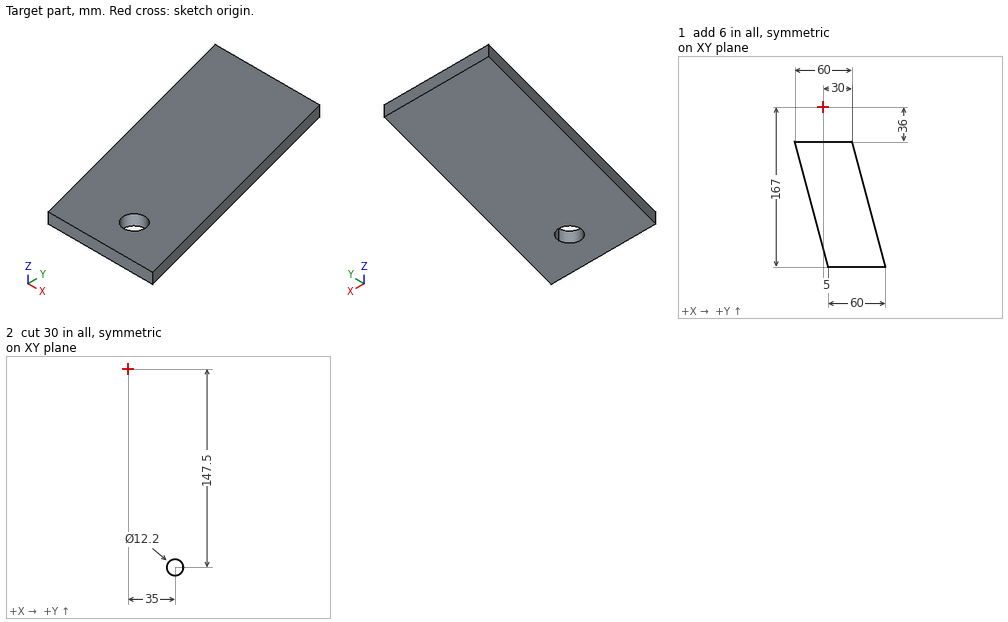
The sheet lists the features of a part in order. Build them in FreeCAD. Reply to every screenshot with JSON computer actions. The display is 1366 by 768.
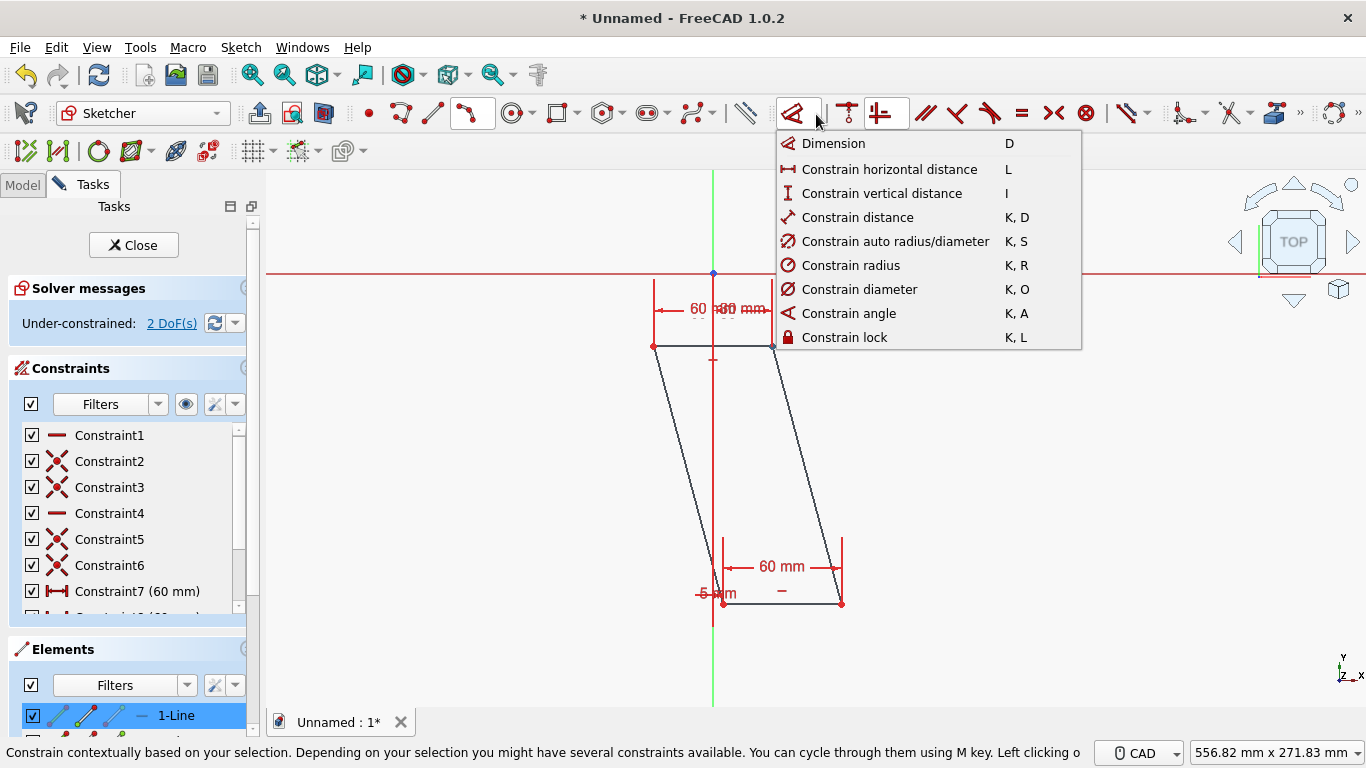
{"action": "left_click", "coordinate": [929, 193]}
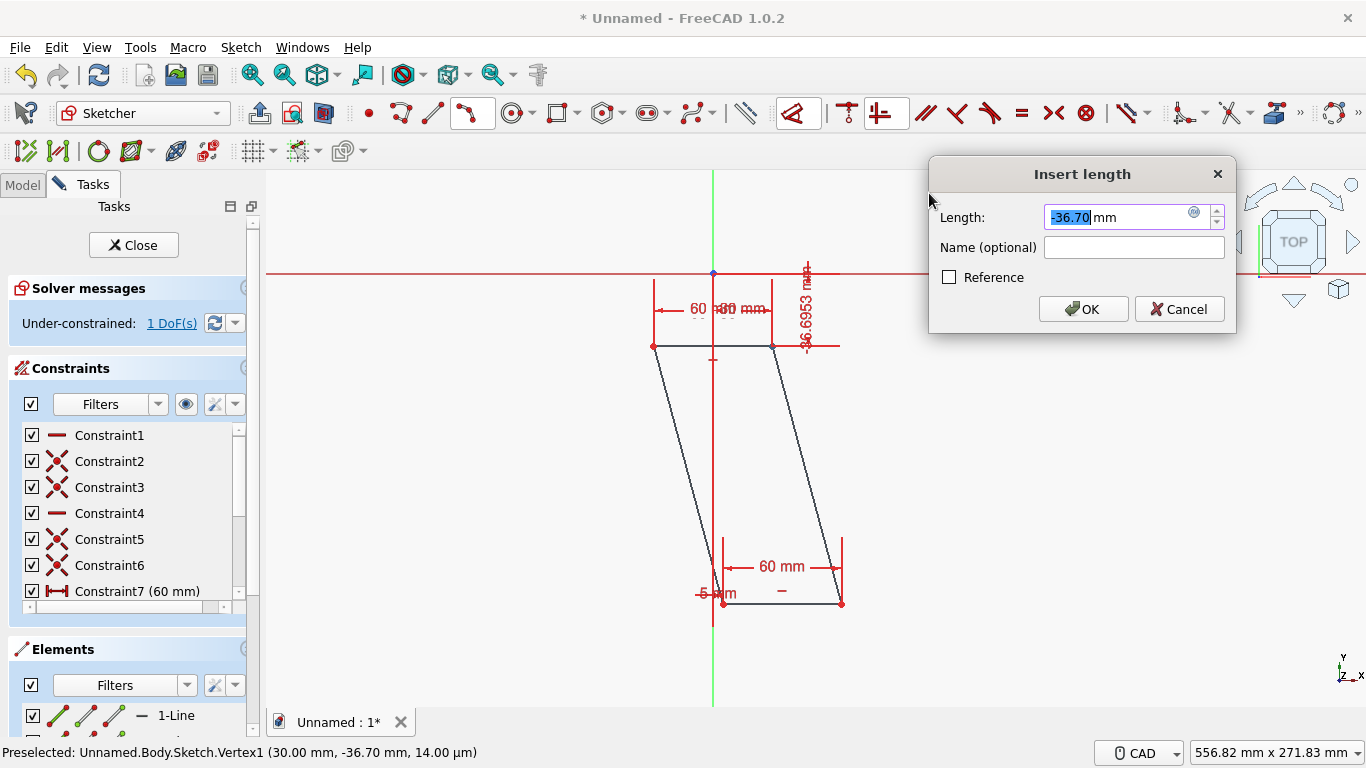
{"action": "type", "text": "-36"}
{"action": "key", "text": "Return"}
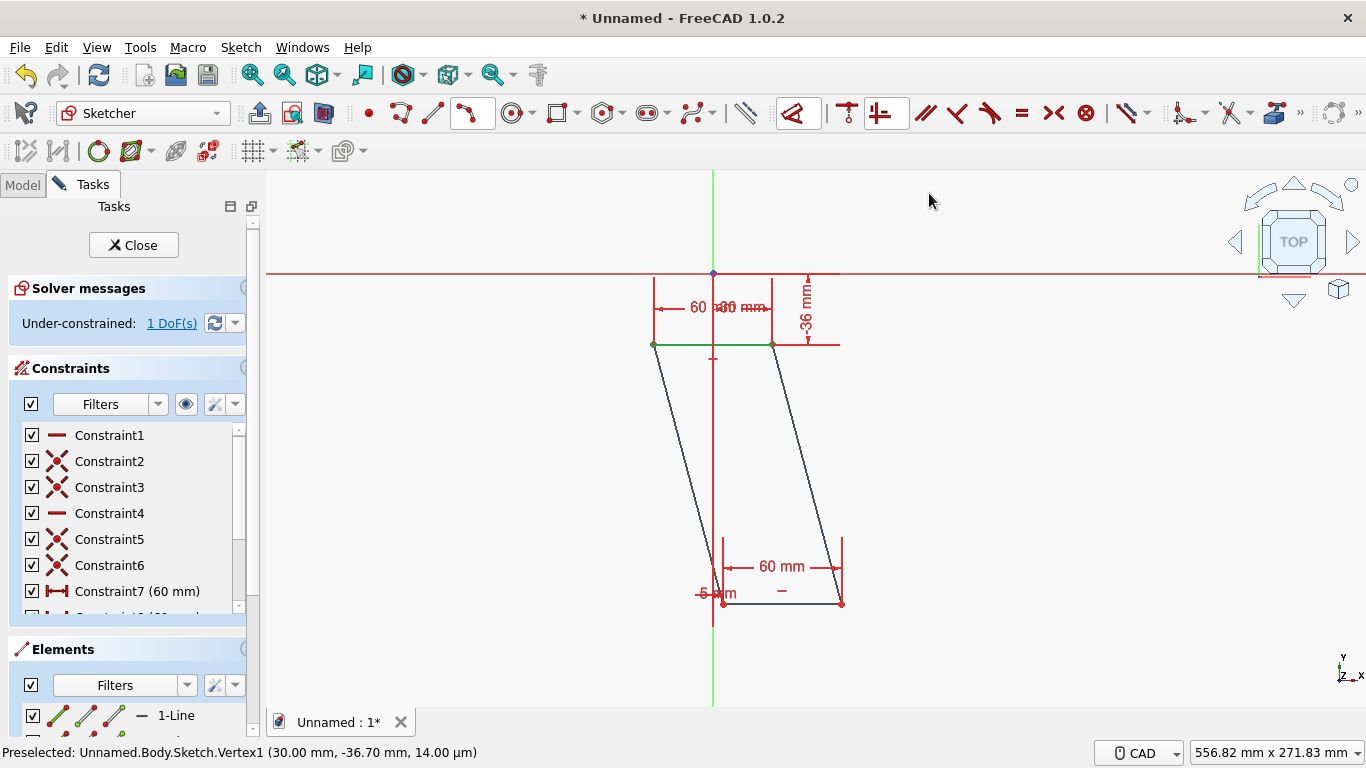
{"action": "left_click", "coordinate": [723, 604]}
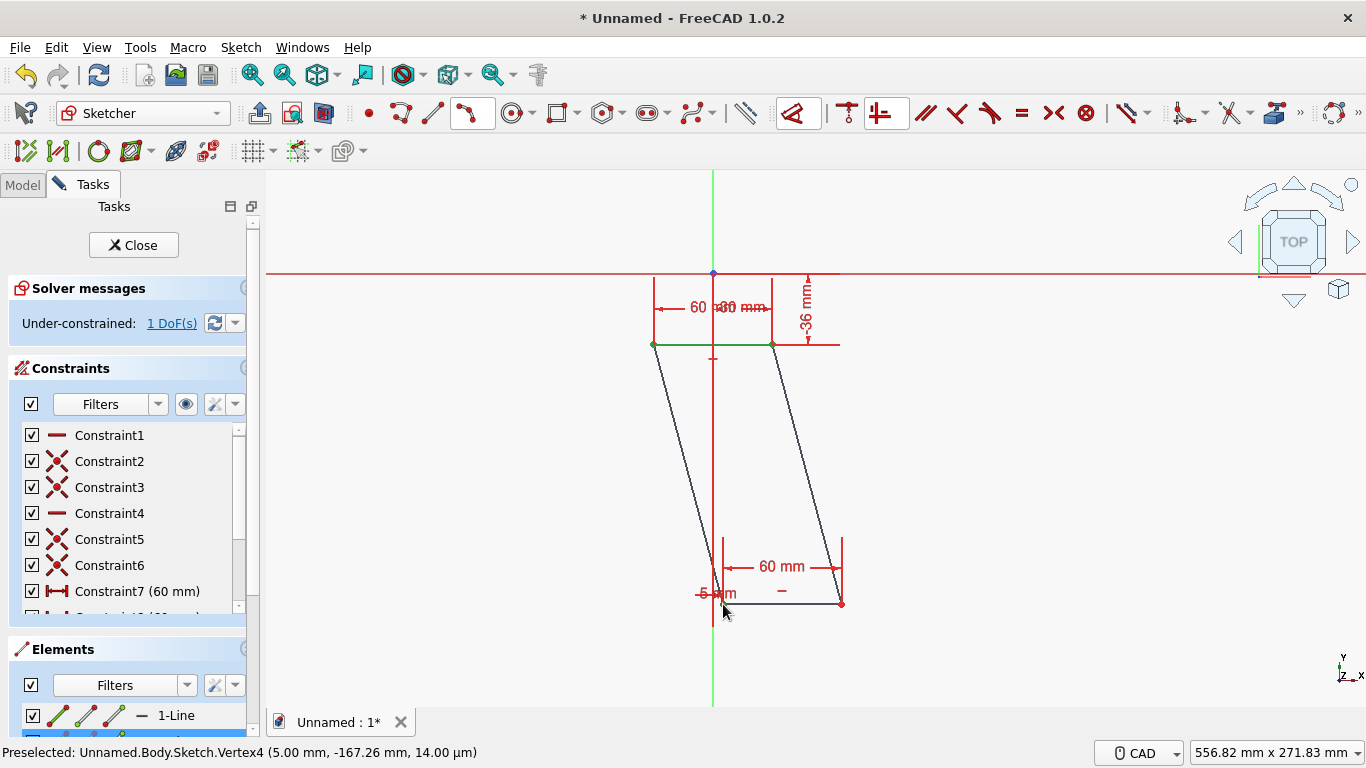
{"action": "key", "text": "i"}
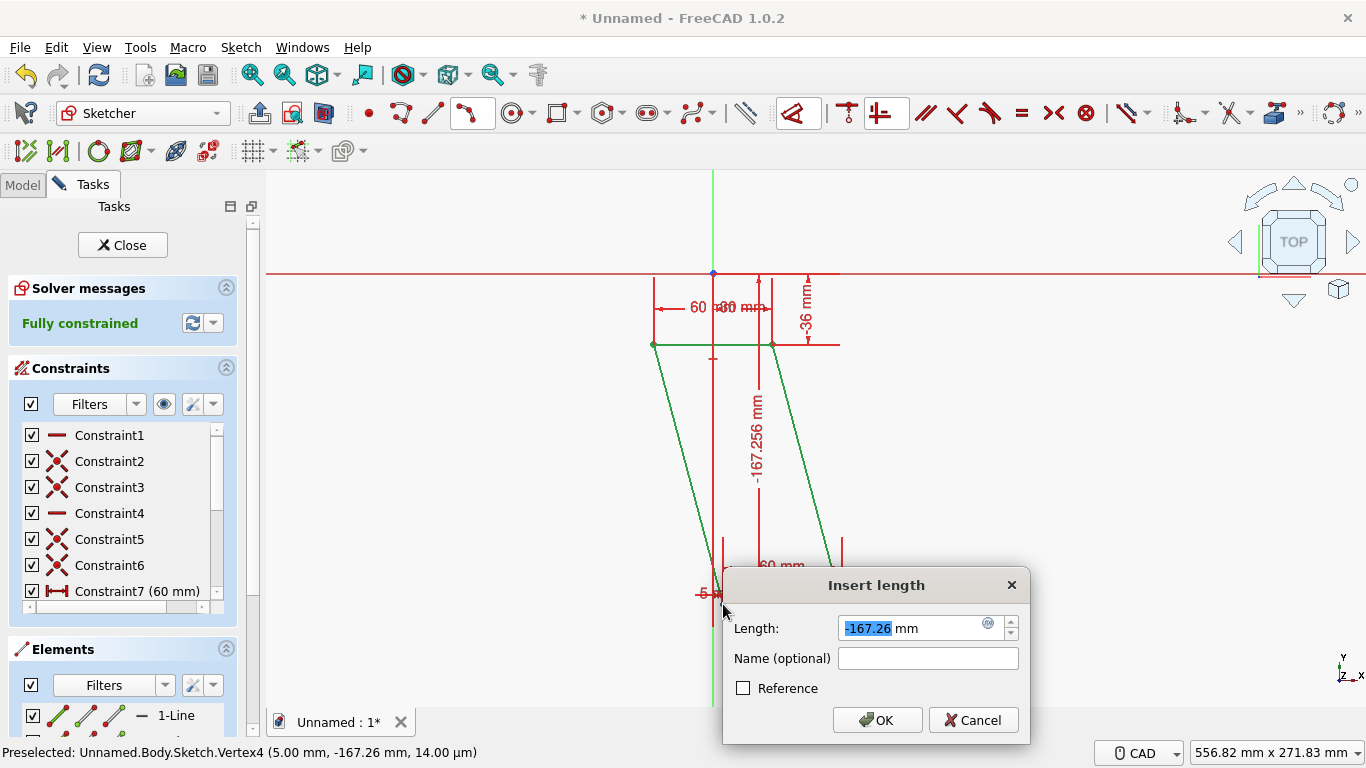
{"action": "type", "text": "-167"}
{"action": "key", "text": "Return"}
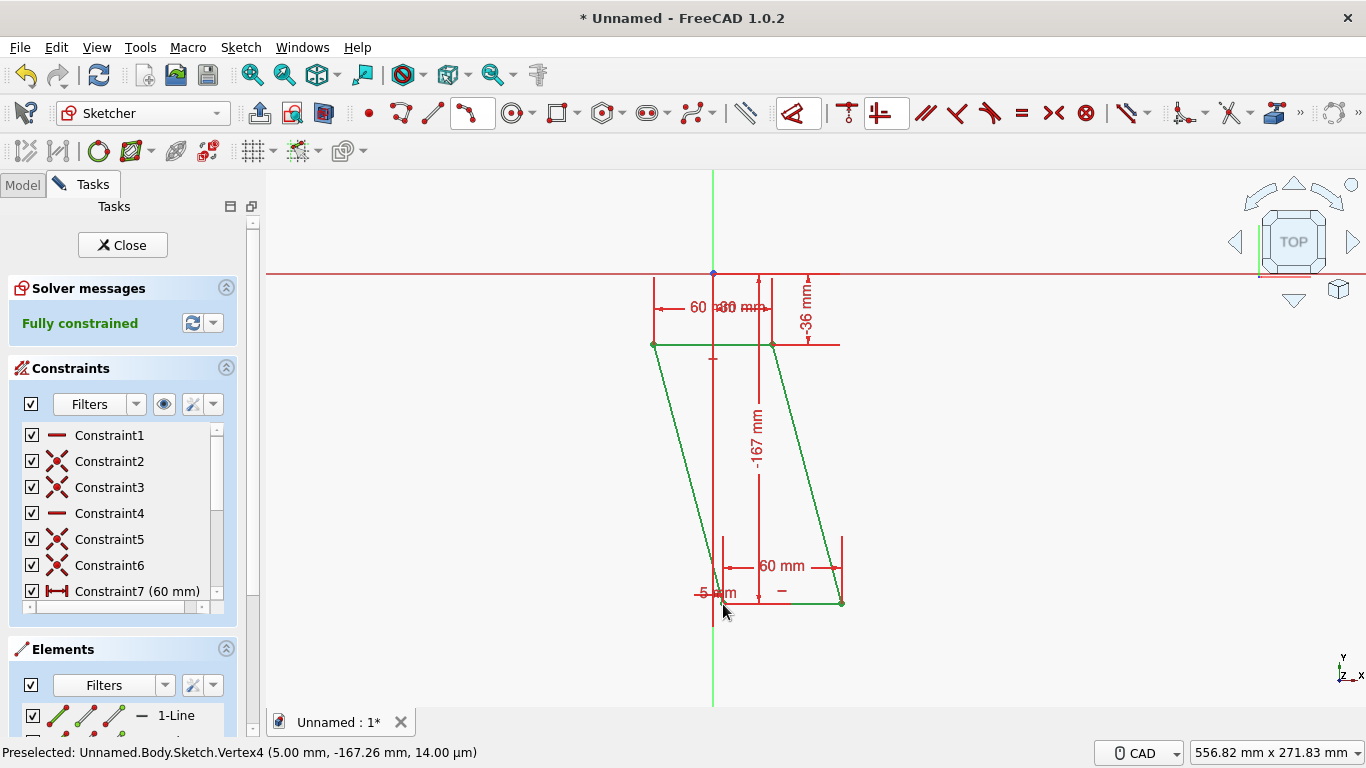
{"action": "left_click", "coordinate": [123, 245]}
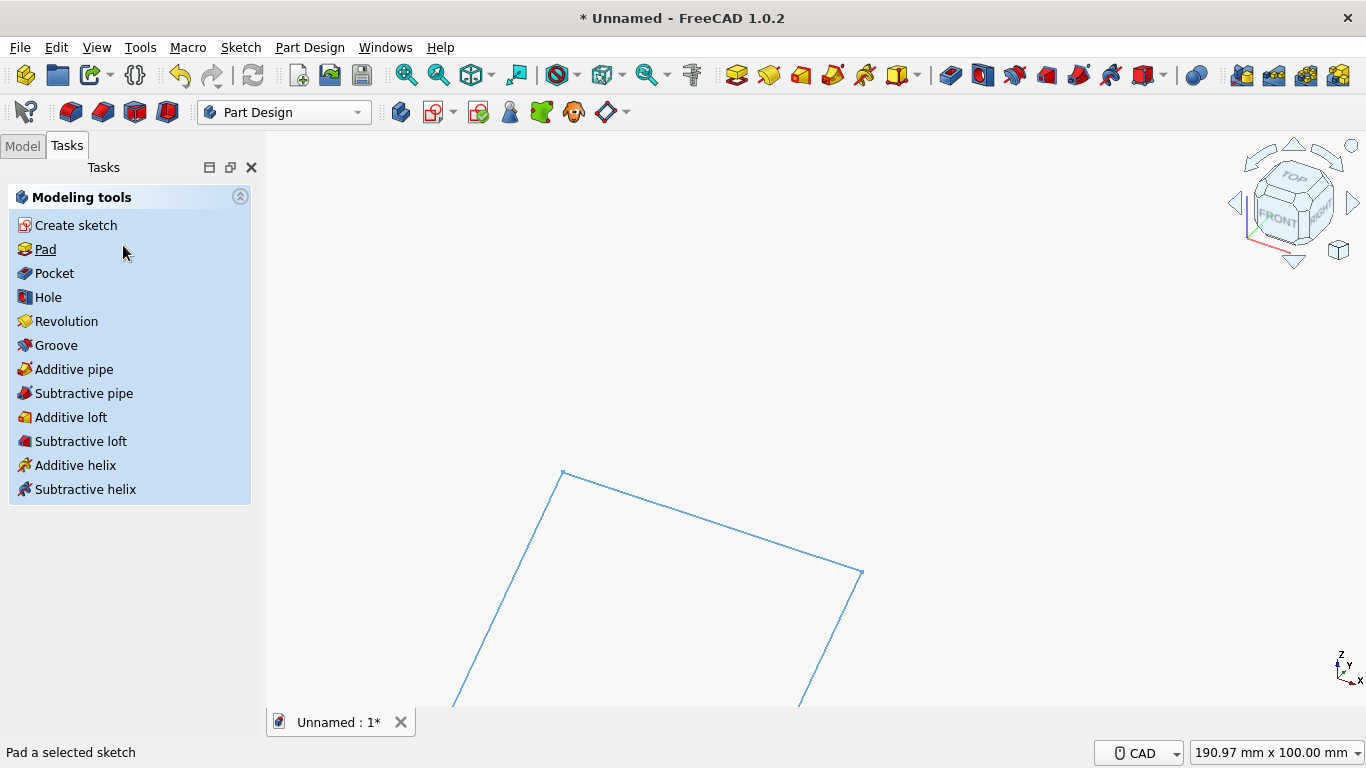
{"action": "left_click", "coordinate": [738, 76]}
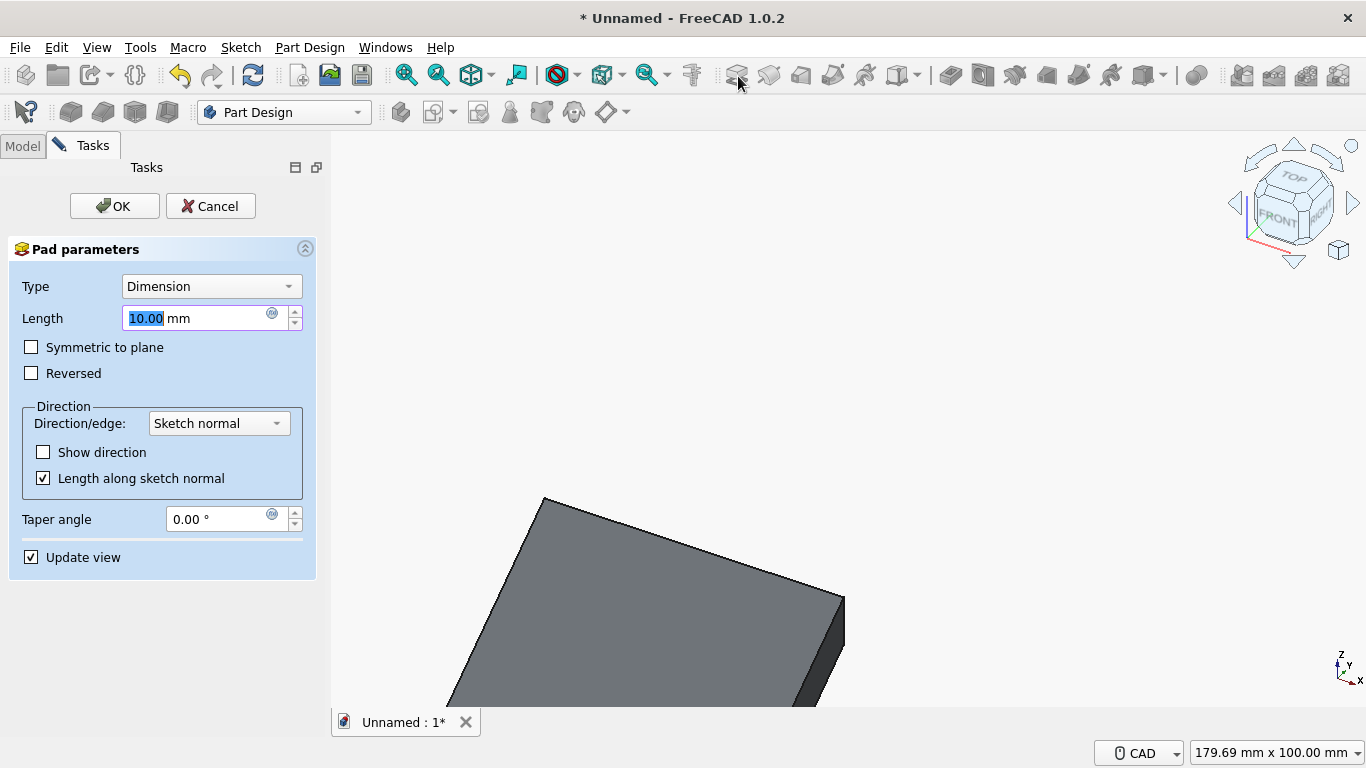
{"action": "type", "text": "6"}
{"action": "key", "text": "Tab"}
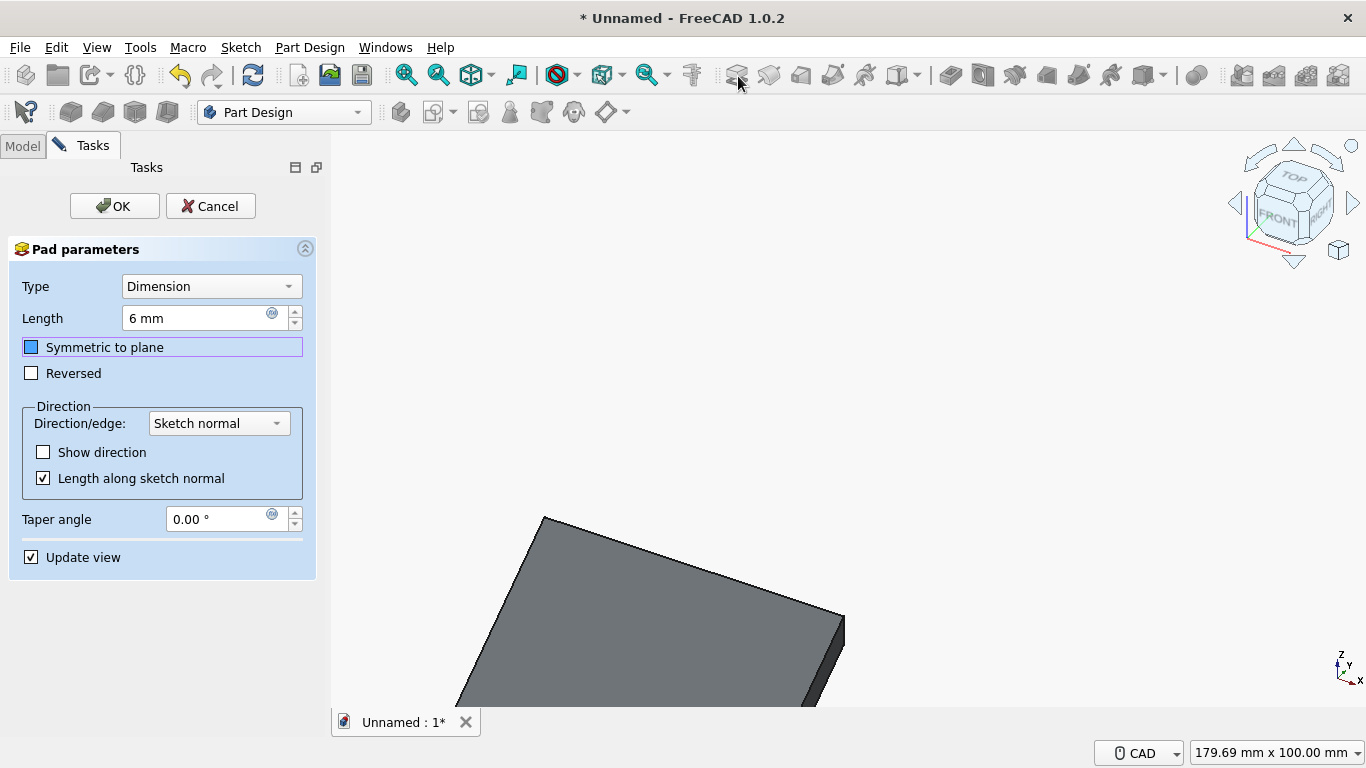
{"action": "left_click", "coordinate": [30, 347]}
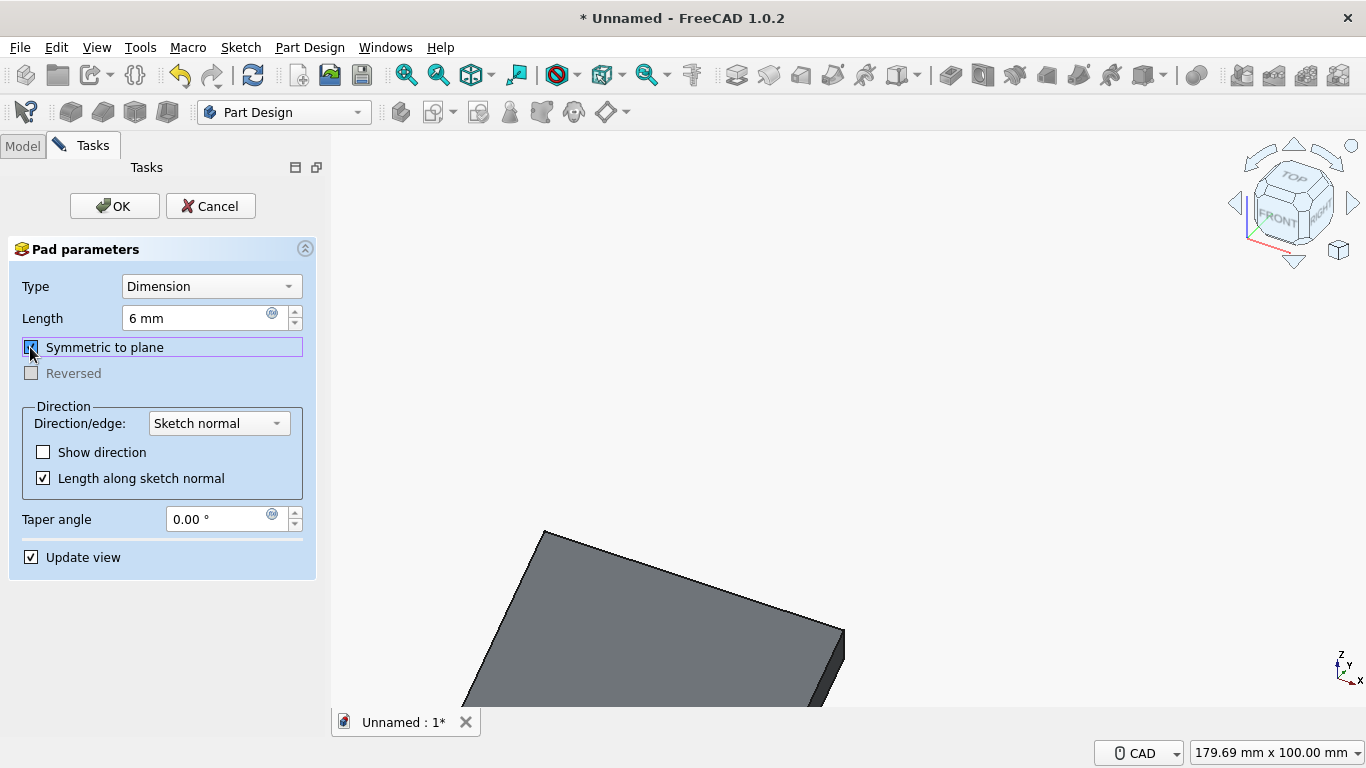
{"action": "left_click", "coordinate": [115, 206]}